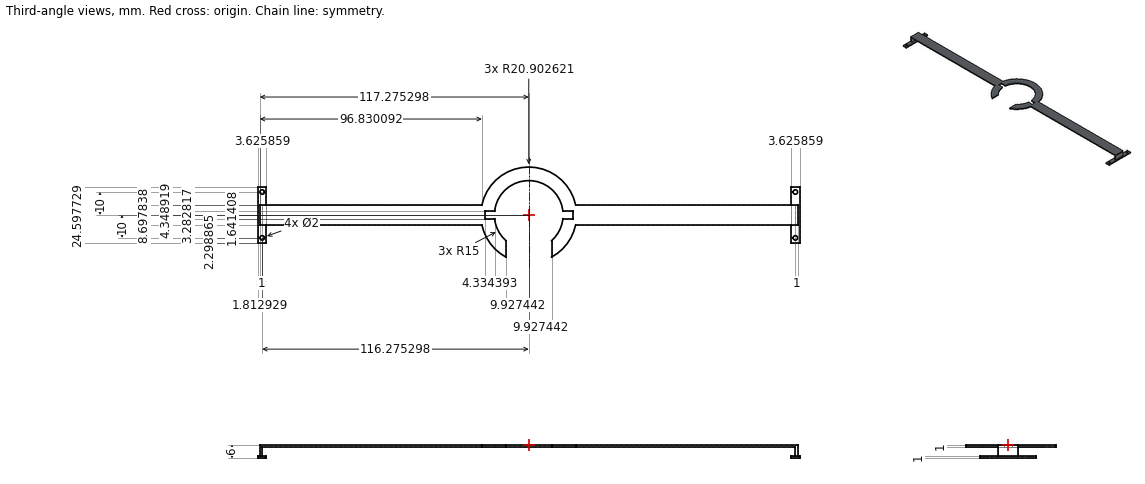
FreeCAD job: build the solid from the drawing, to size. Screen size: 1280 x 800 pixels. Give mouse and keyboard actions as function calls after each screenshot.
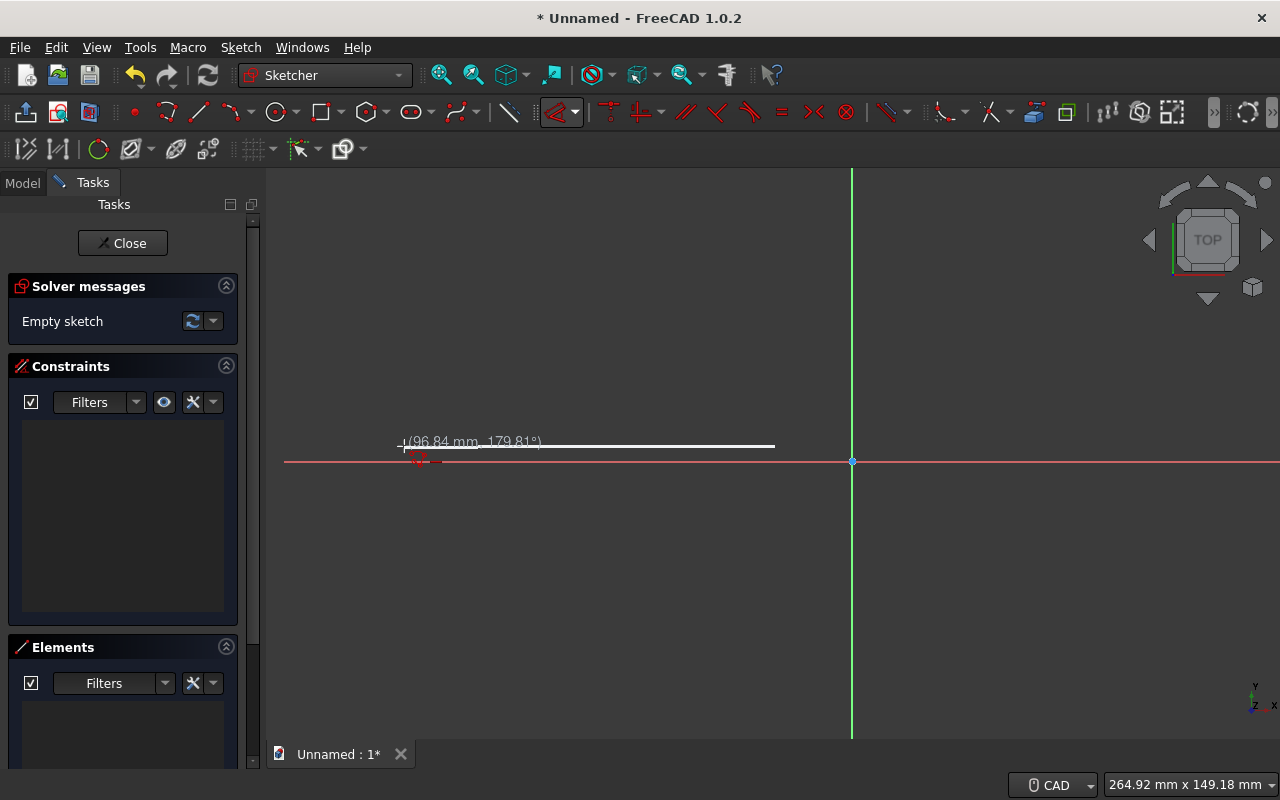
click(403, 445)
click(403, 479)
click(774, 479)
right_click(774, 479)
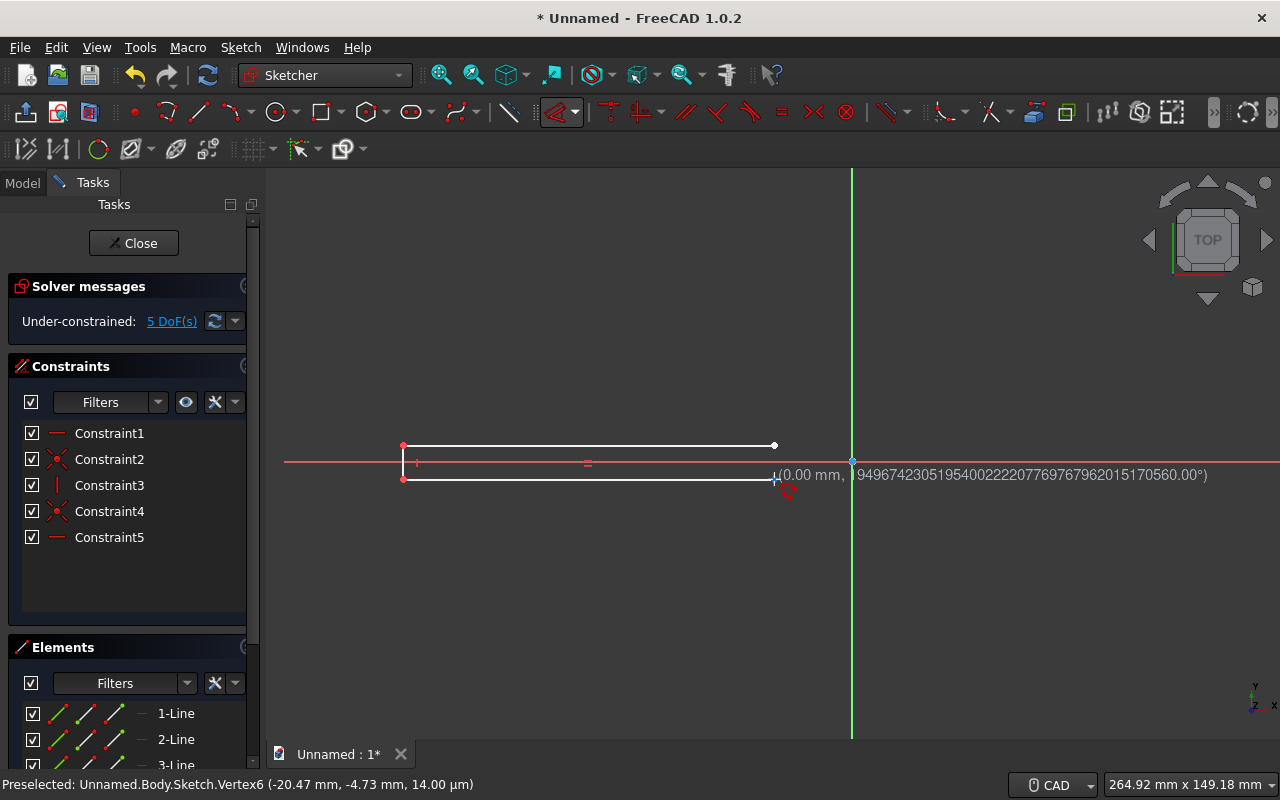
click(200, 112)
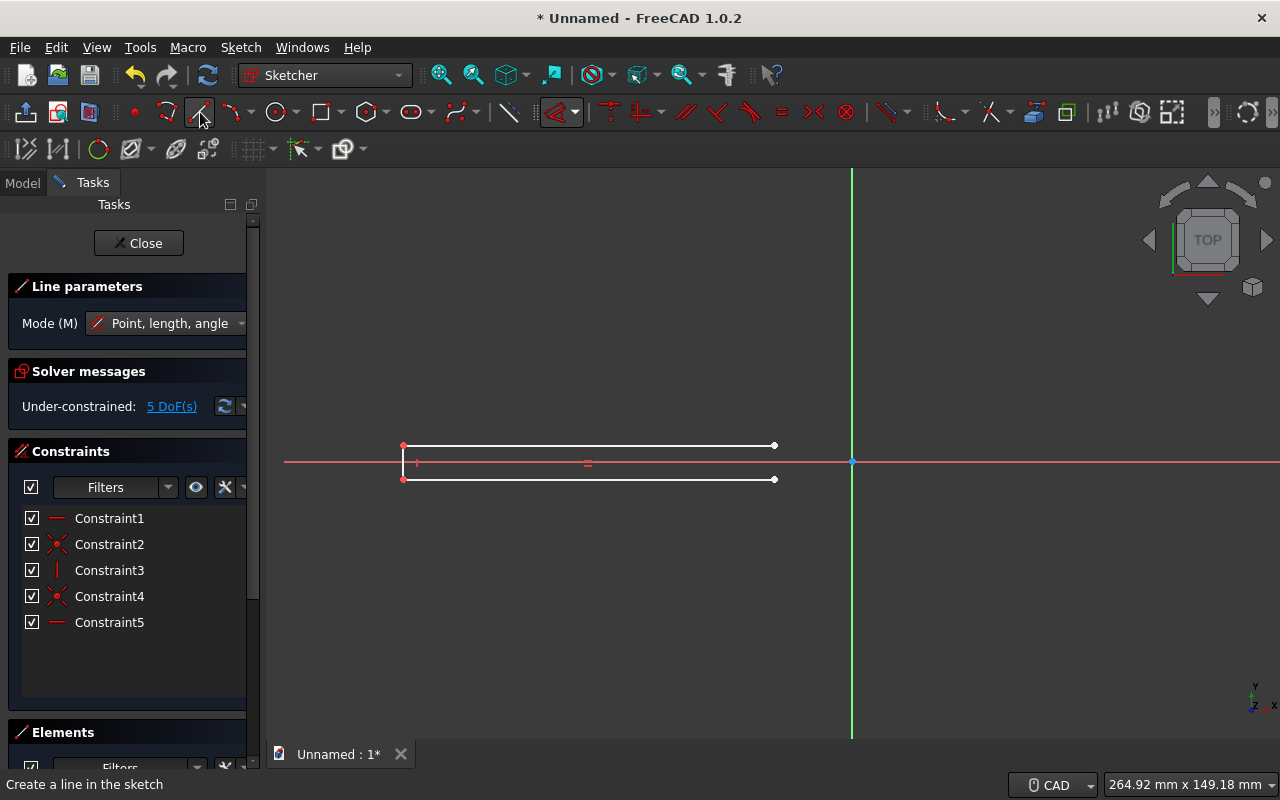
click(814, 532)
click(814, 505)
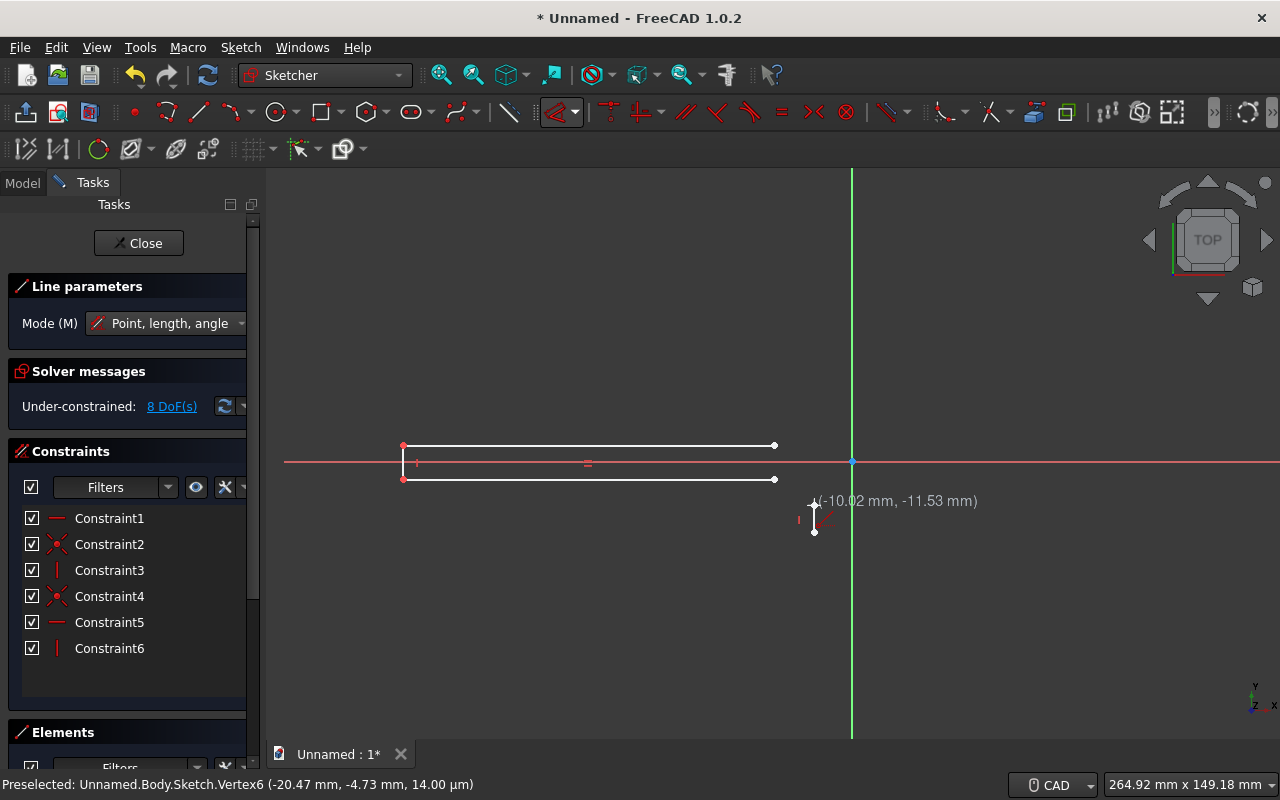
click(168, 112)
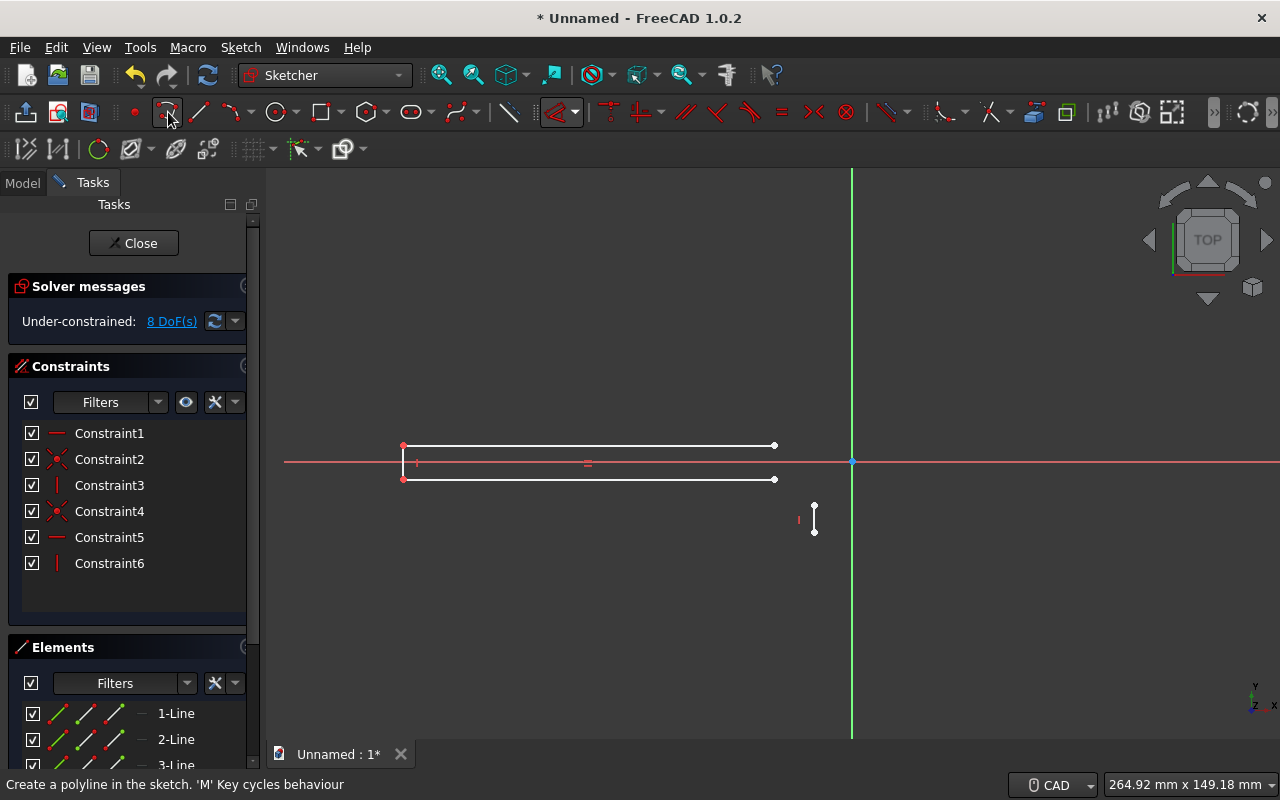
scroll(795, 468, up, 5)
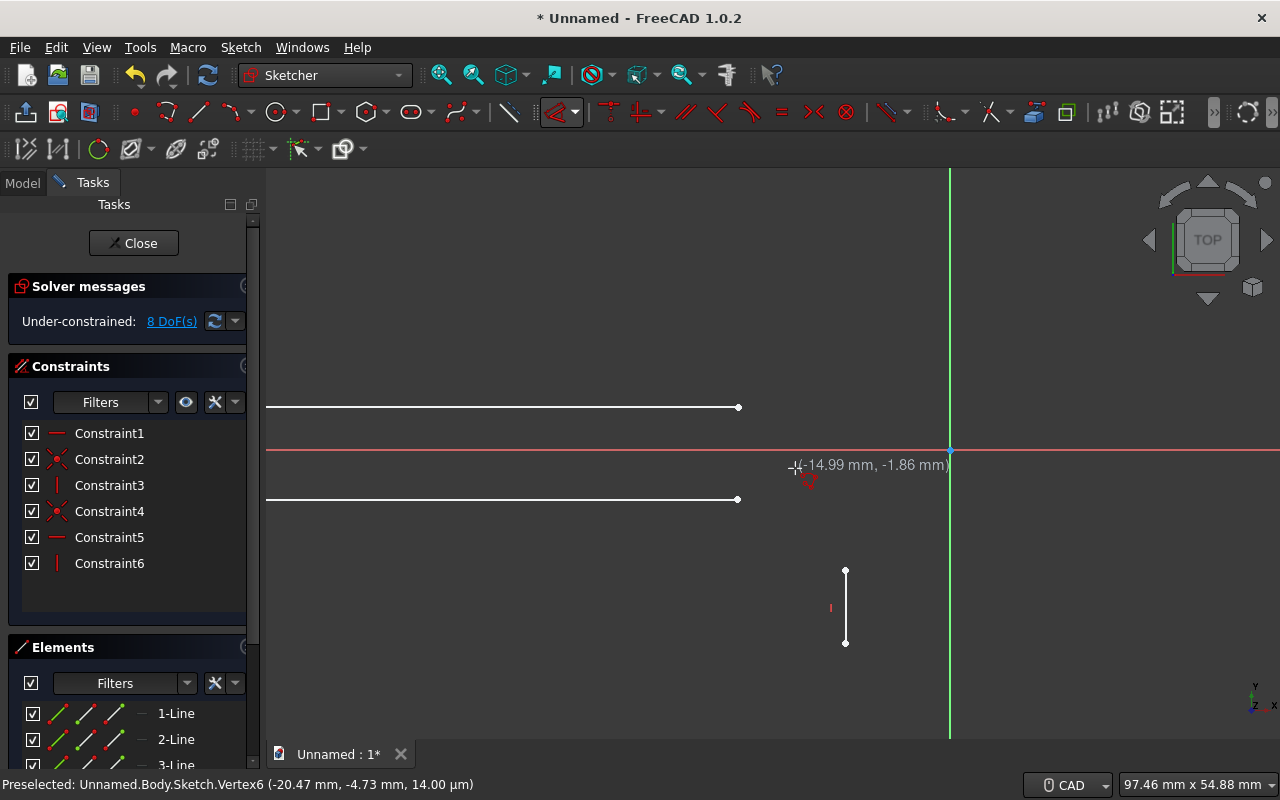
click(795, 468)
click(750, 468)
click(750, 433)
click(795, 433)
right_click(795, 433)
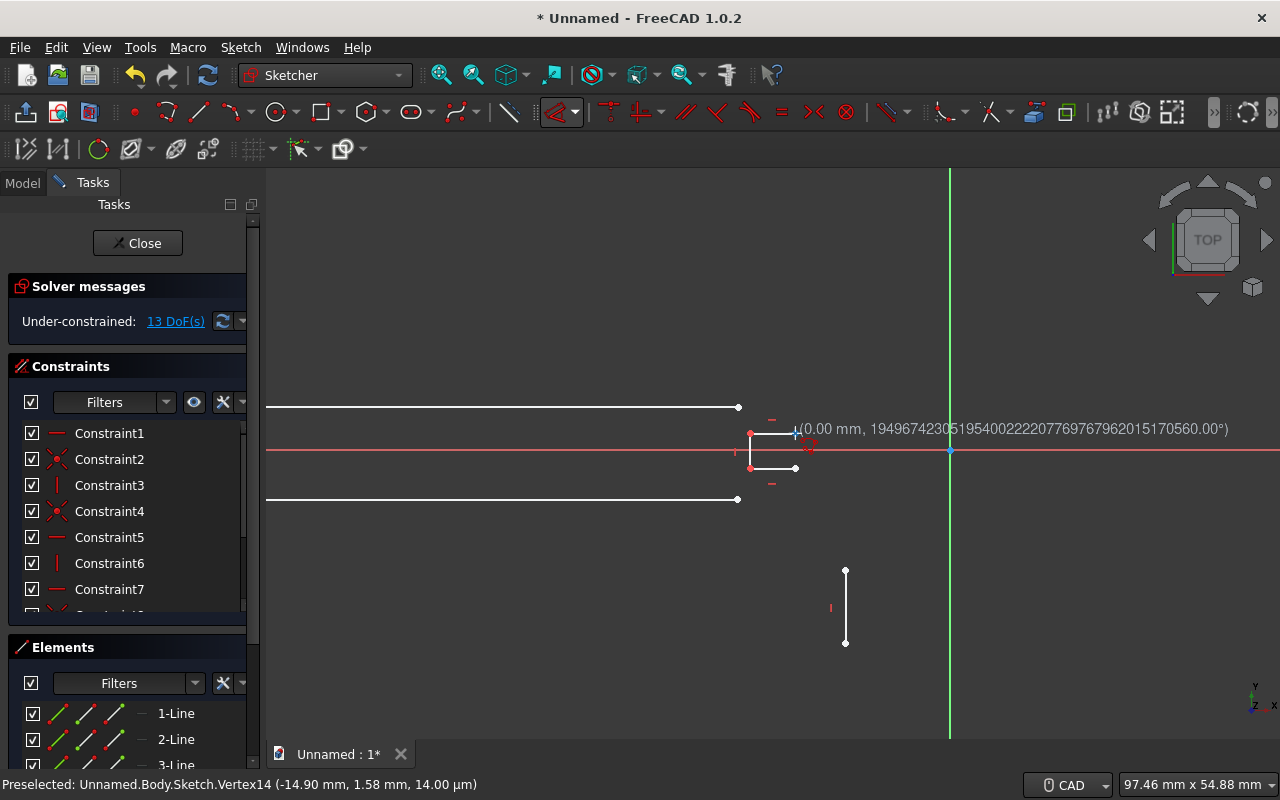
click(1105, 433)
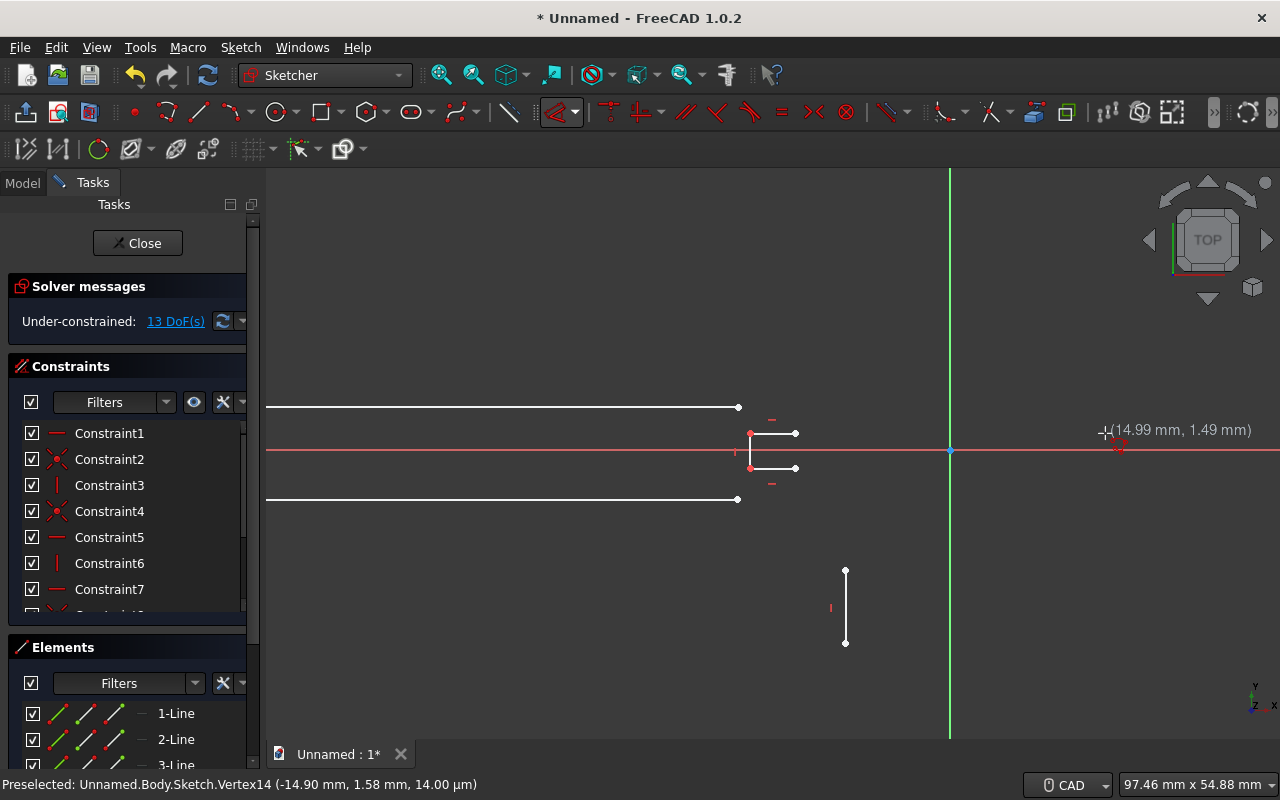
scroll(624, 459, down, 7)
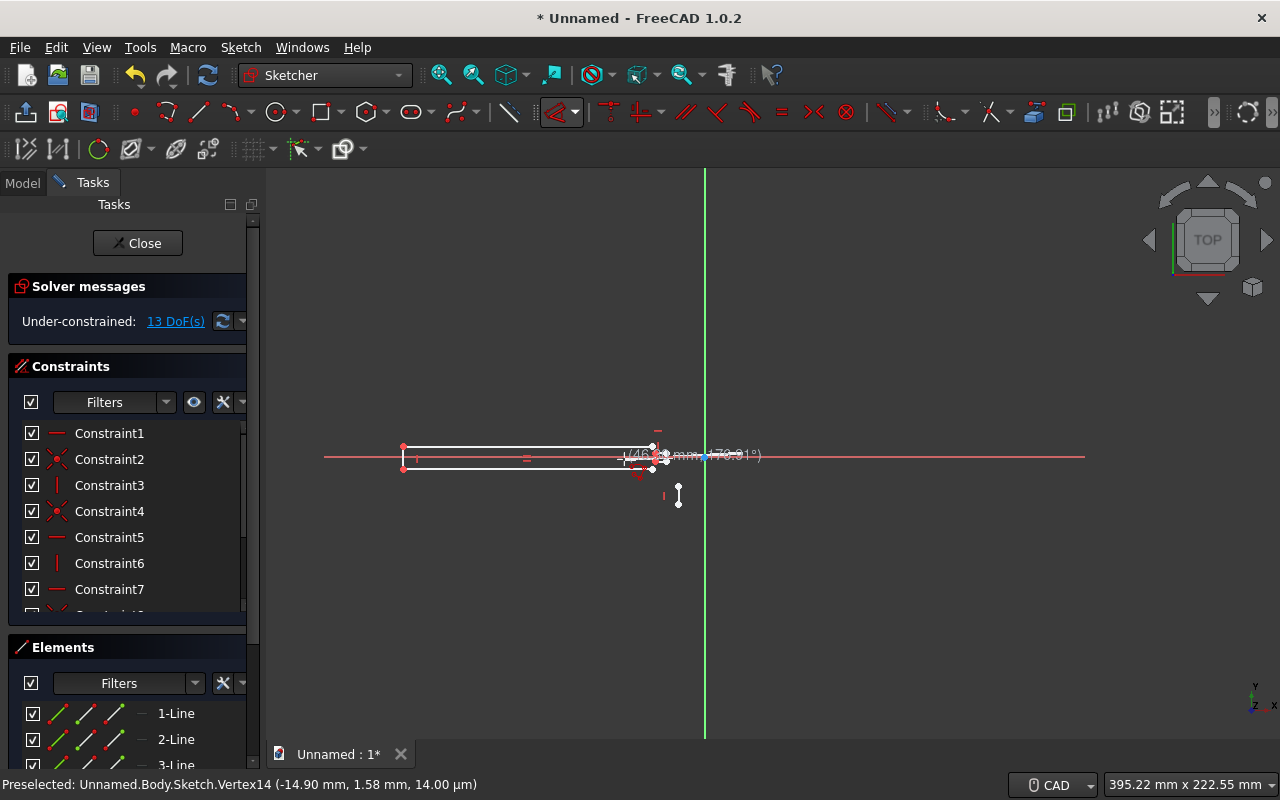
scroll(754, 453, up, 7)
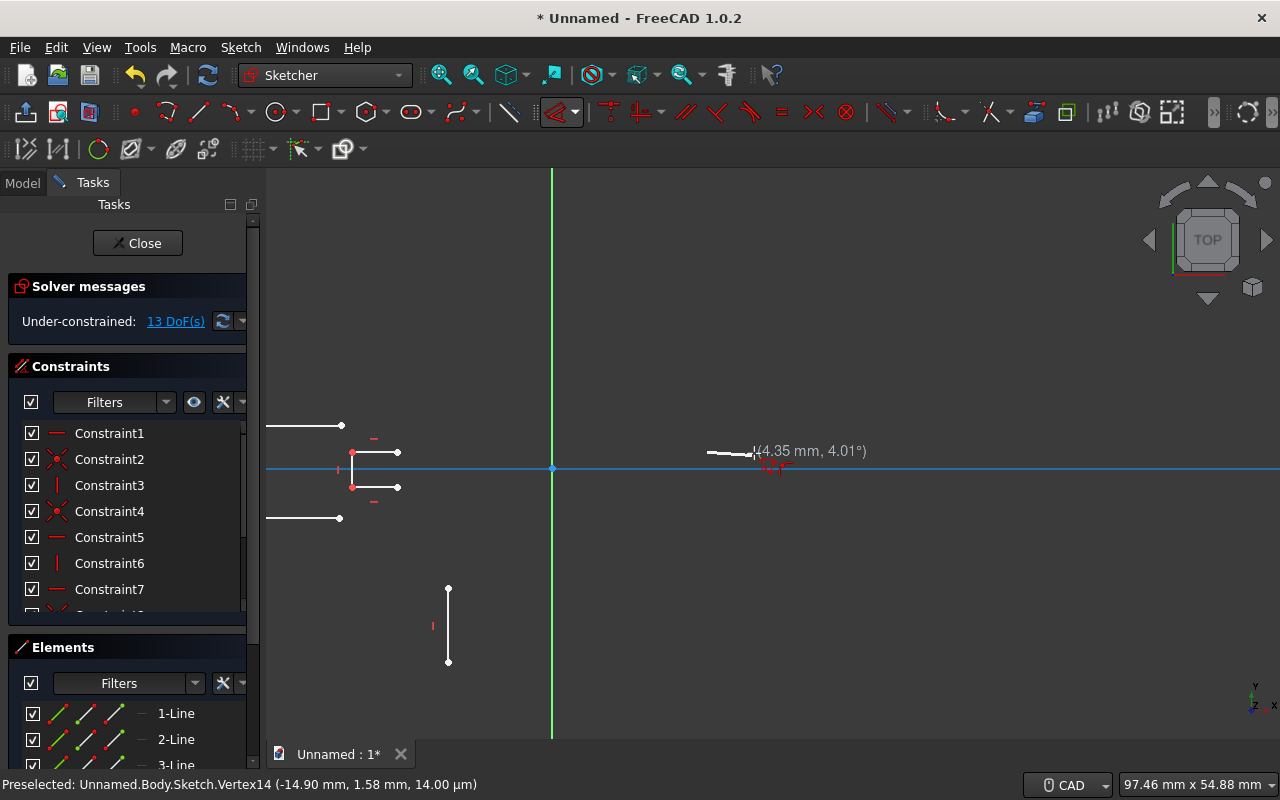
click(753, 451)
click(753, 486)
click(708, 486)
right_click(708, 486)